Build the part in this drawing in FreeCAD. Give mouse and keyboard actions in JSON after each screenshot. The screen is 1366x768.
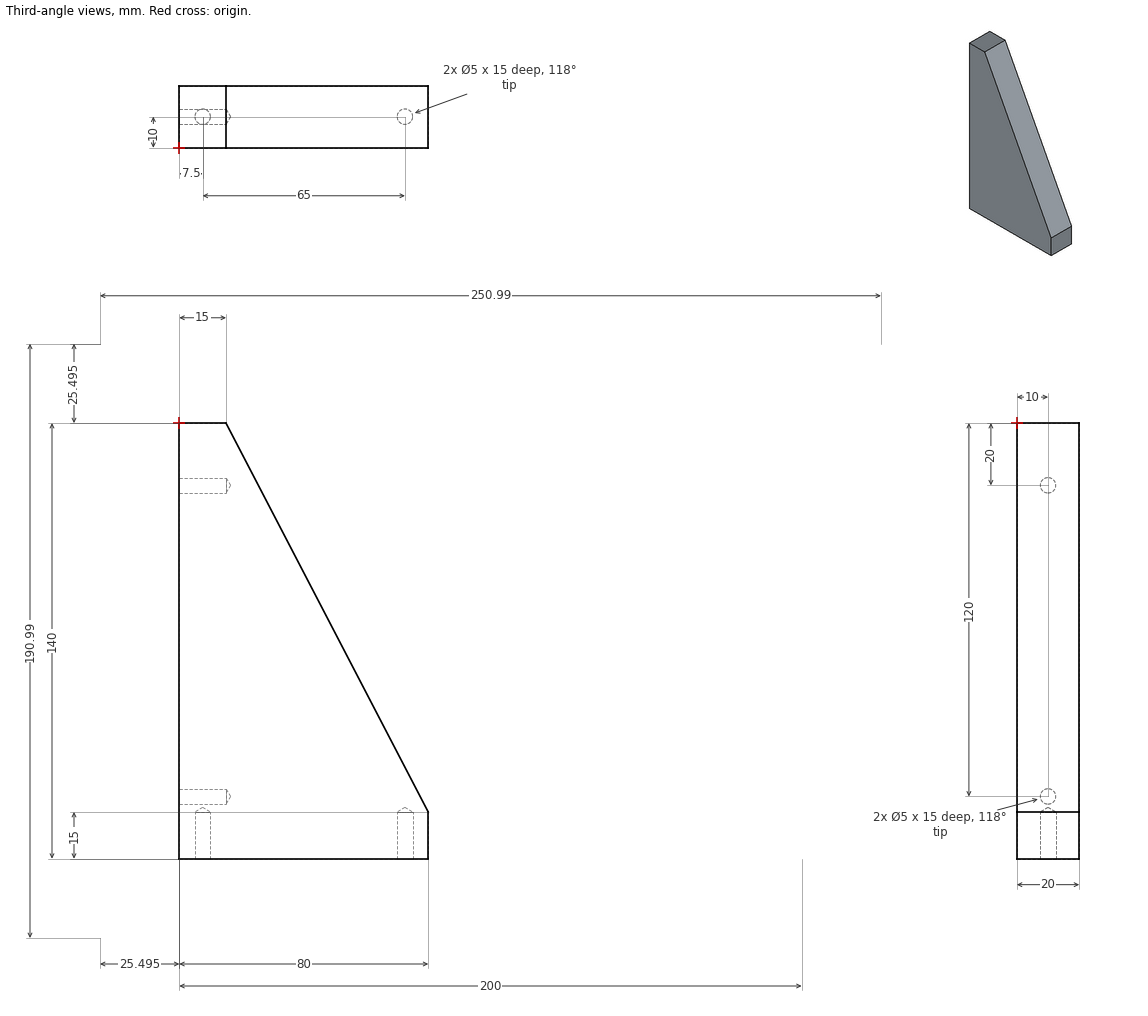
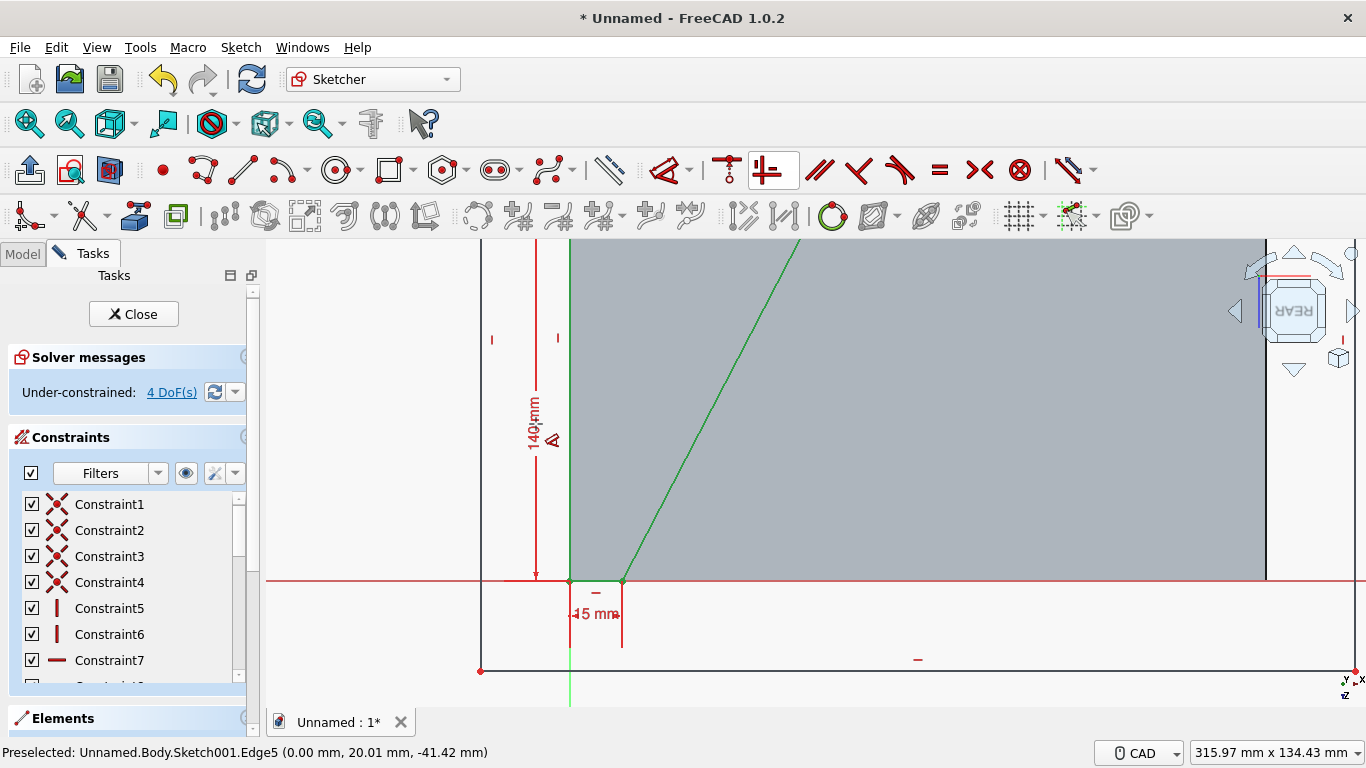
{"action": "left_click", "coordinate": [481, 472]}
{"action": "left_click", "coordinate": [447, 469]}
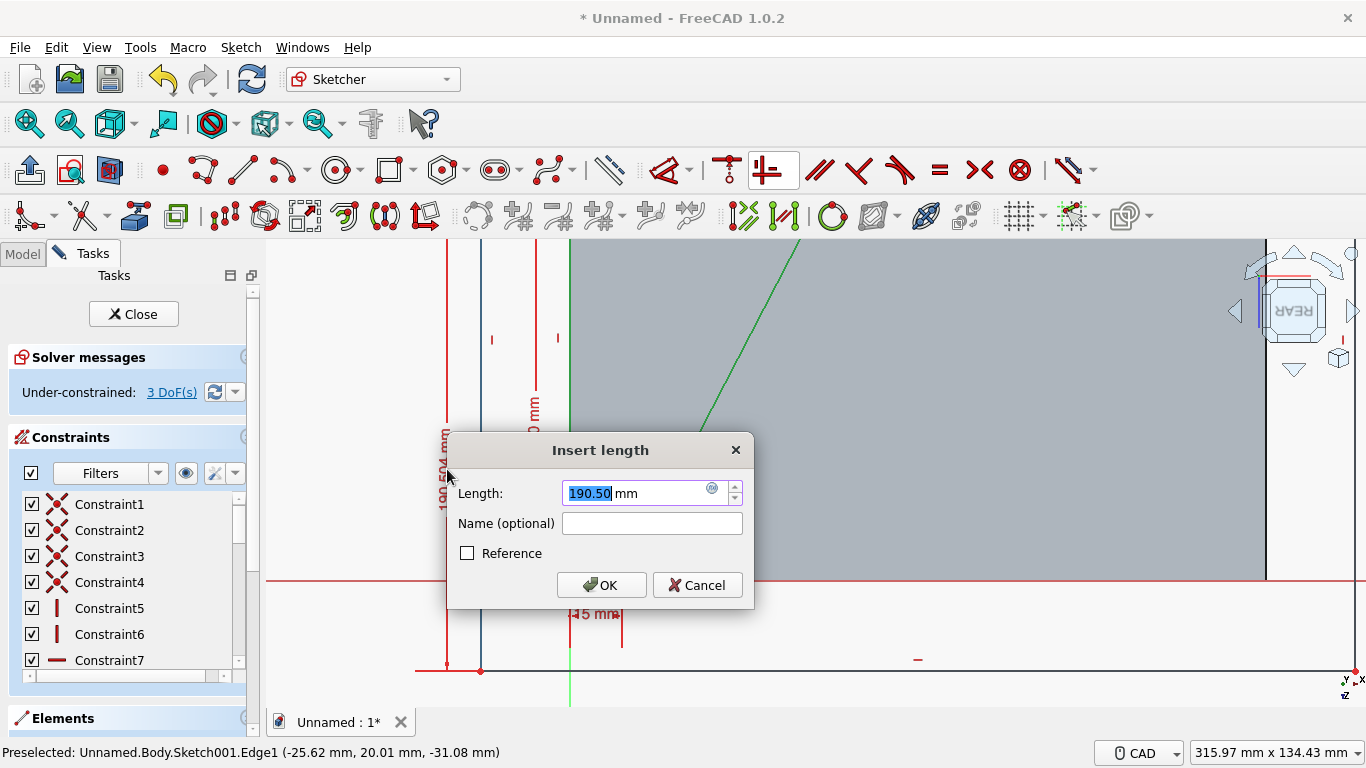
{"action": "type", "text": "190.99"}
{"action": "key", "text": "Return"}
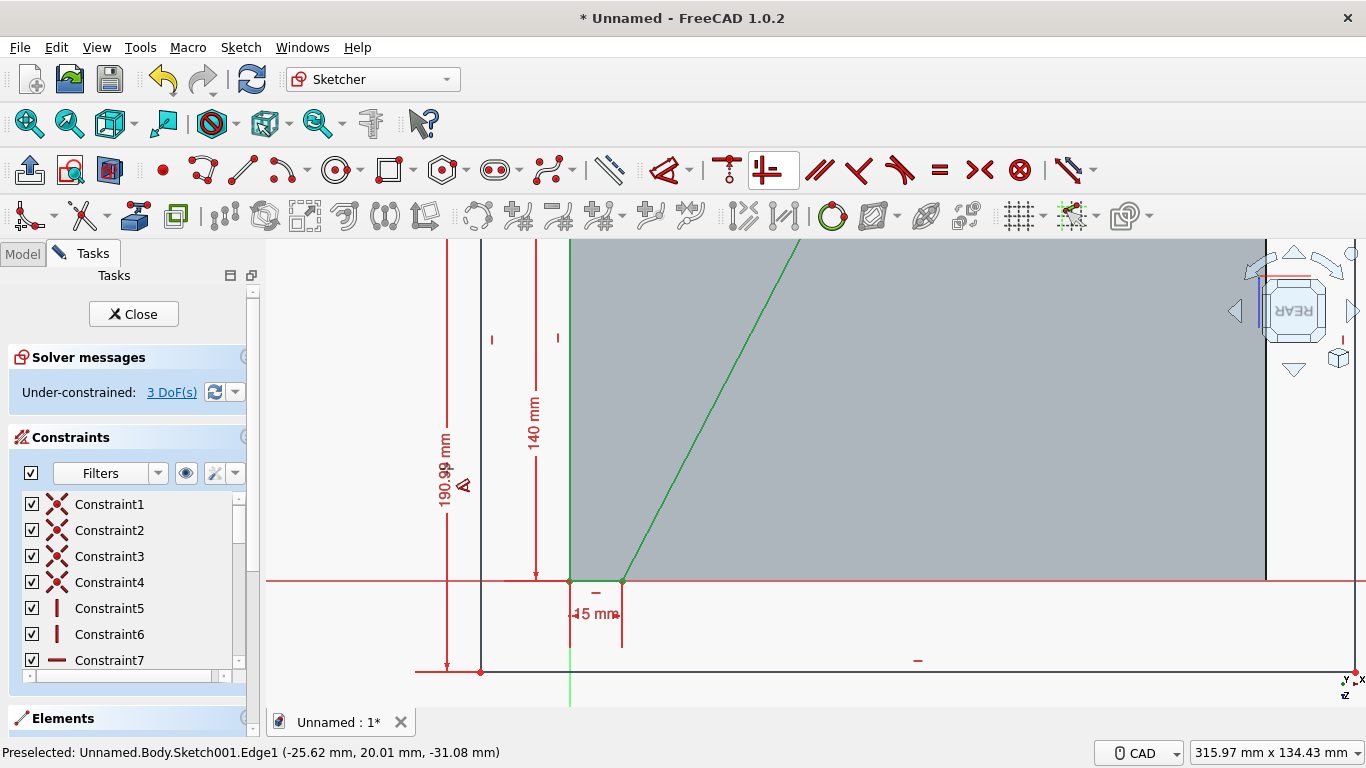
{"action": "left_click", "coordinate": [743, 672]}
{"action": "left_click", "coordinate": [841, 638]}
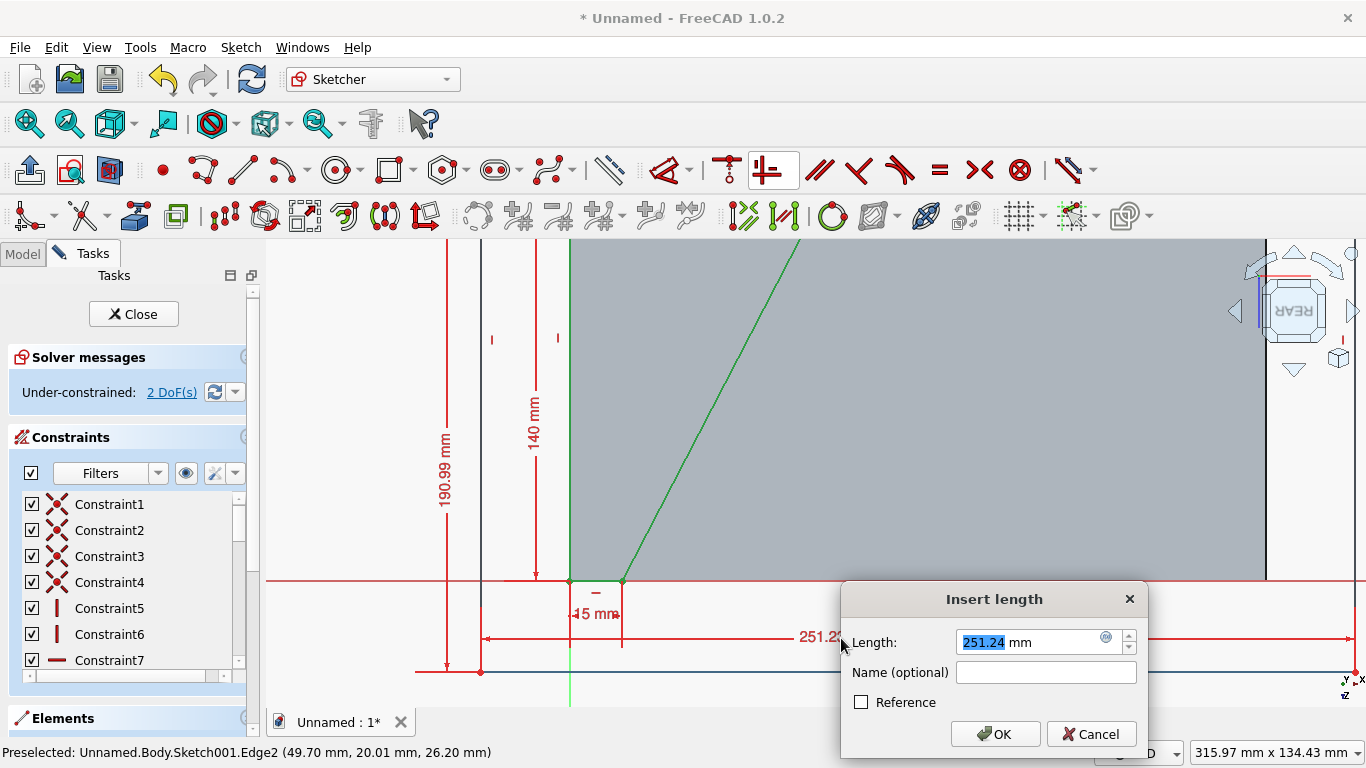
{"action": "type", "text": "250.99"}
{"action": "key", "text": "Return"}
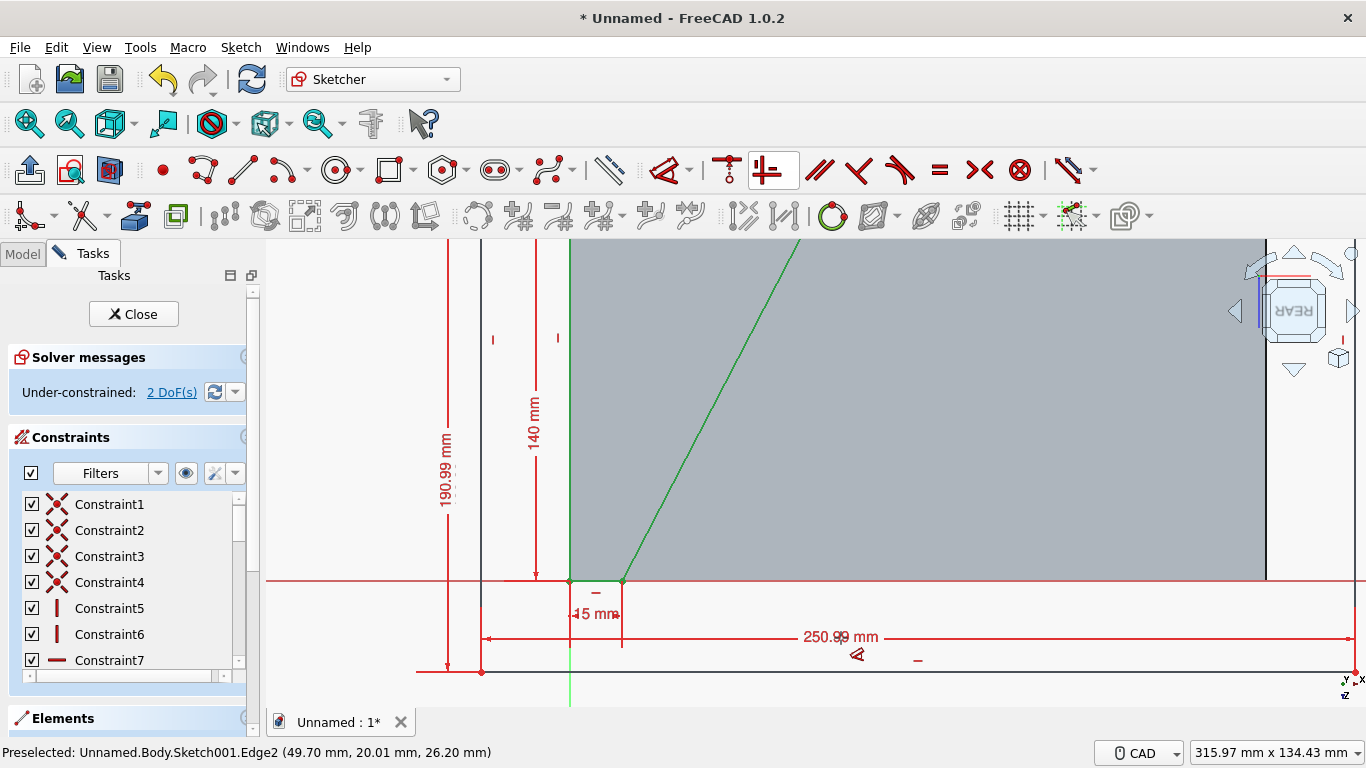
{"action": "scroll", "coordinate": [608, 584], "scroll_direction": "down", "scroll_amount": 4}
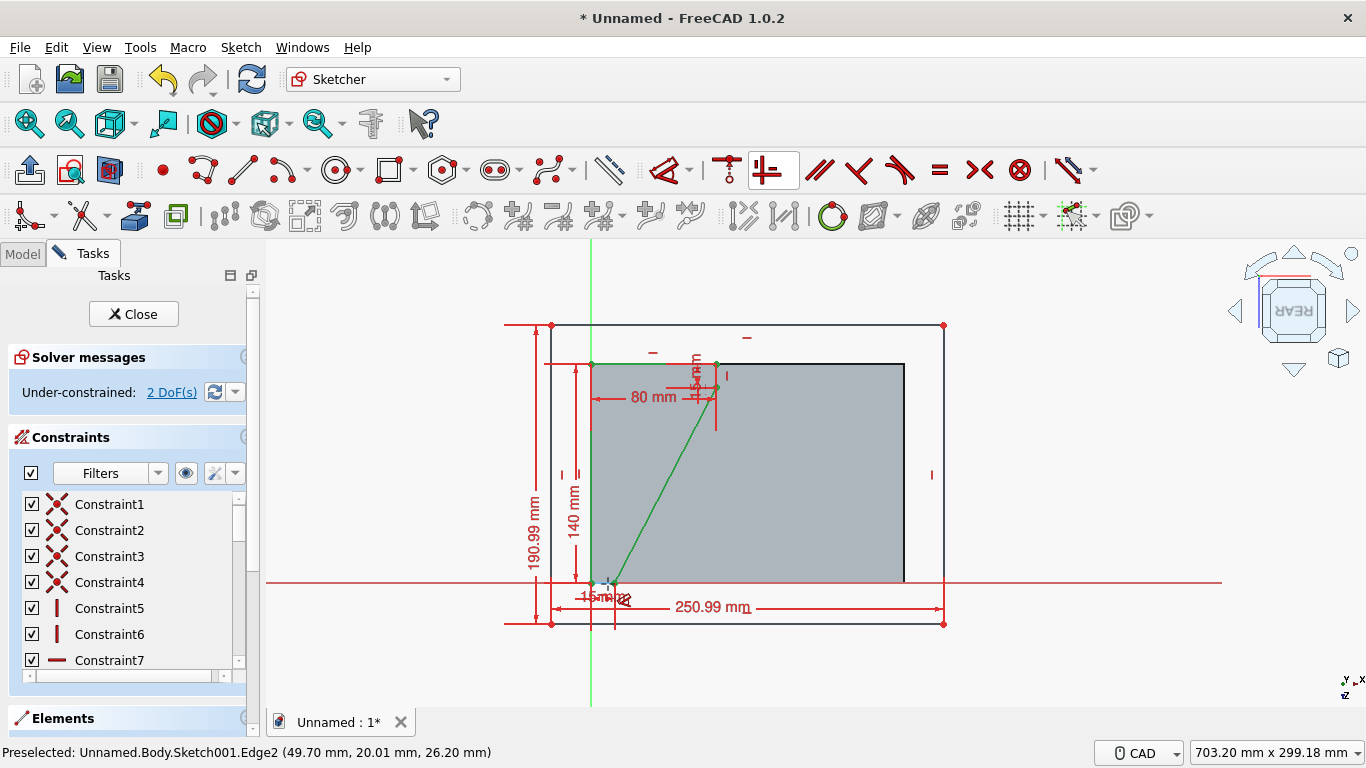
{"action": "left_click", "coordinate": [551, 325]}
{"action": "left_click", "coordinate": [571, 291]}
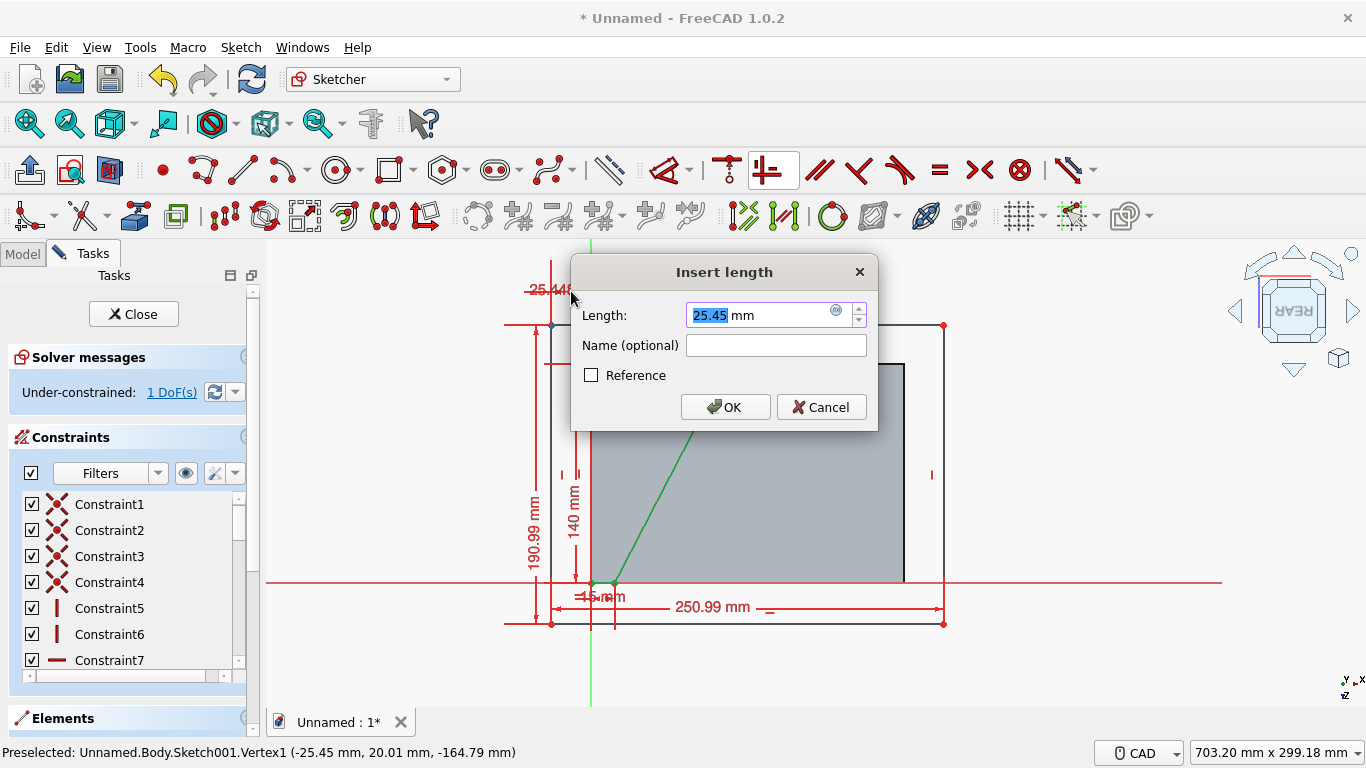
{"action": "type", "text": "25.495"}
{"action": "key", "text": "Return"}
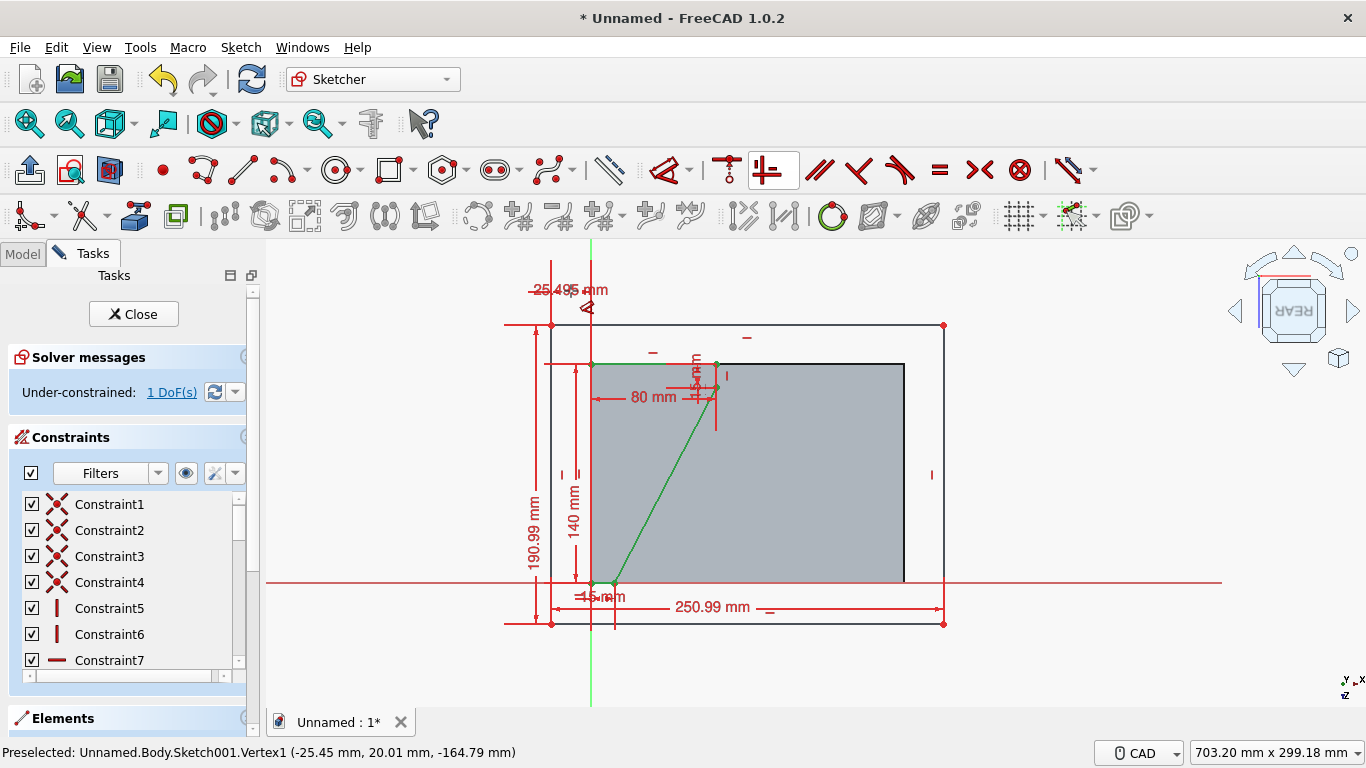
{"action": "left_click", "coordinate": [551, 624]}
{"action": "left_click", "coordinate": [517, 604]}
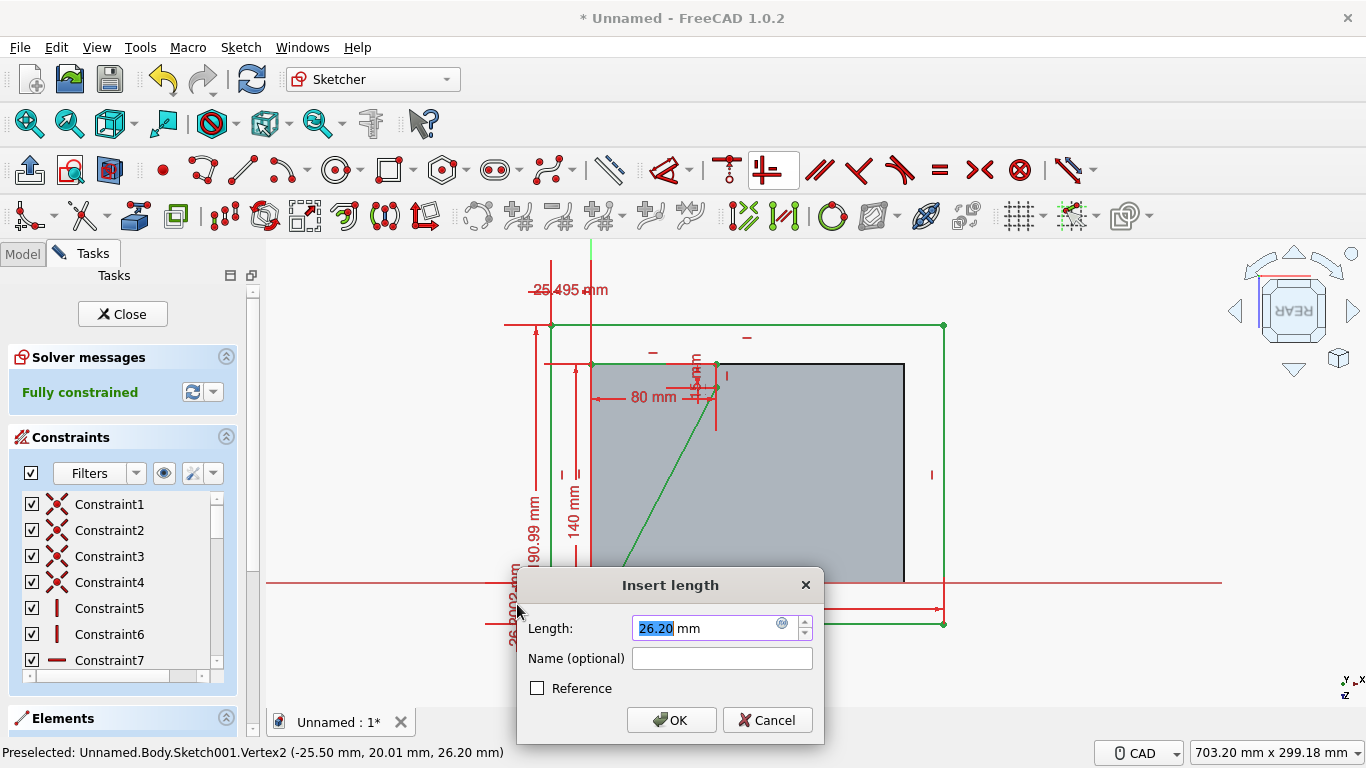
{"action": "type", "text": "25.495"}
{"action": "key", "text": "Return"}
{"action": "key", "text": "Escape"}